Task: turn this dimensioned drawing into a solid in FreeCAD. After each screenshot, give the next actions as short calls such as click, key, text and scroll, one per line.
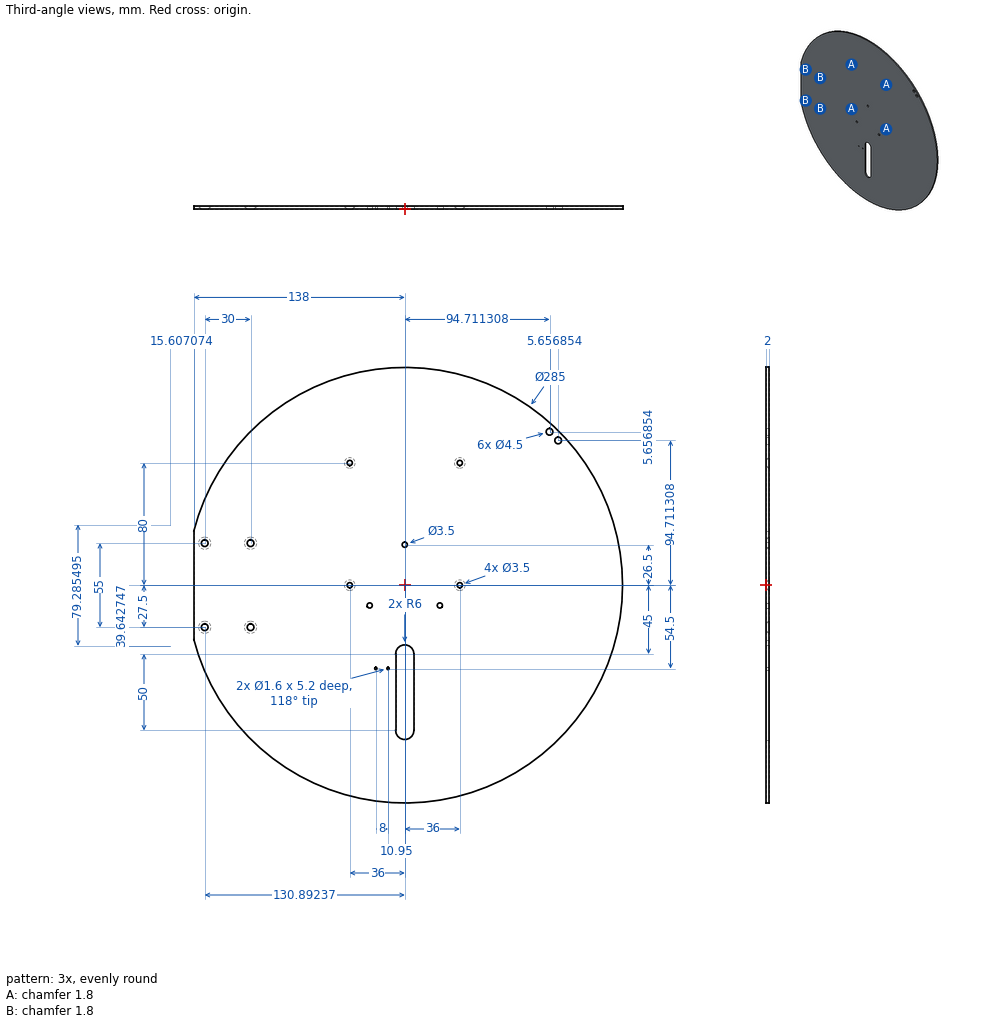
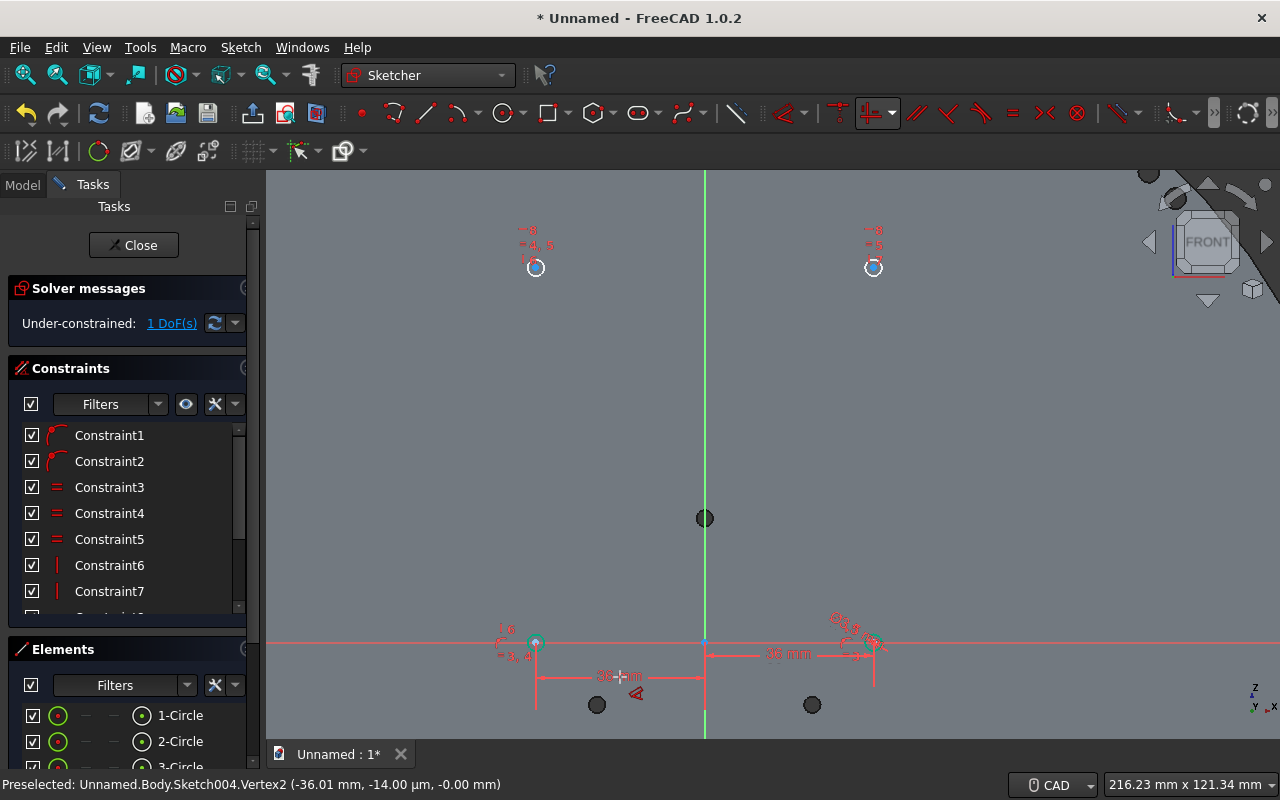
click(536, 268)
click(502, 455)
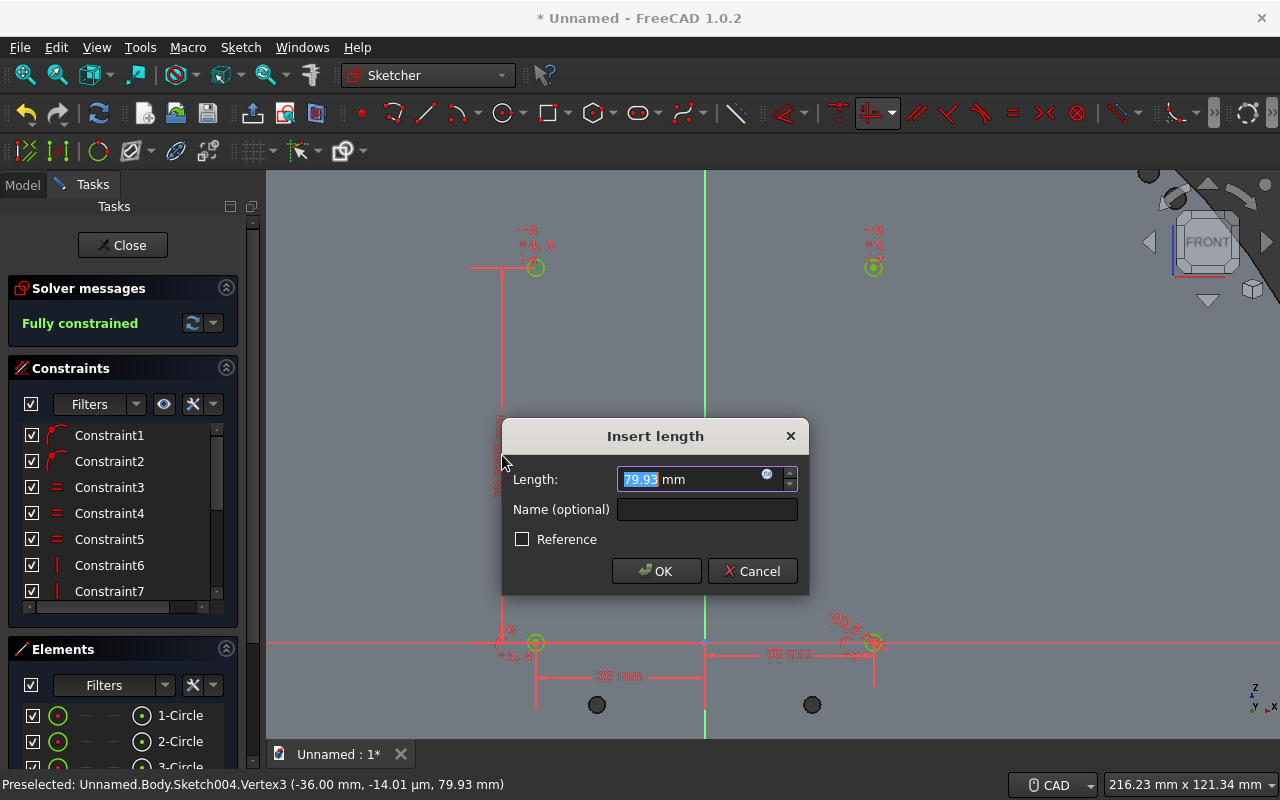
text(80)
key(Return)
key(Escape)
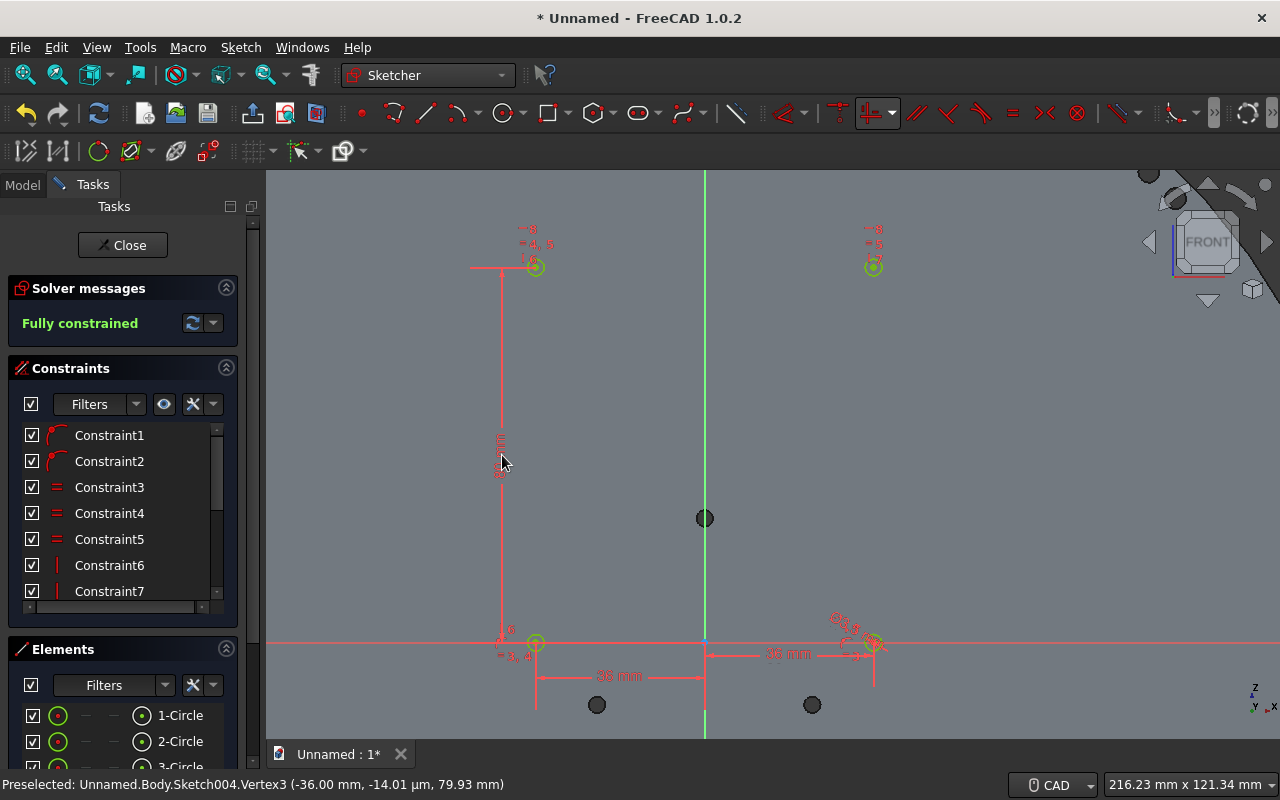
click(123, 245)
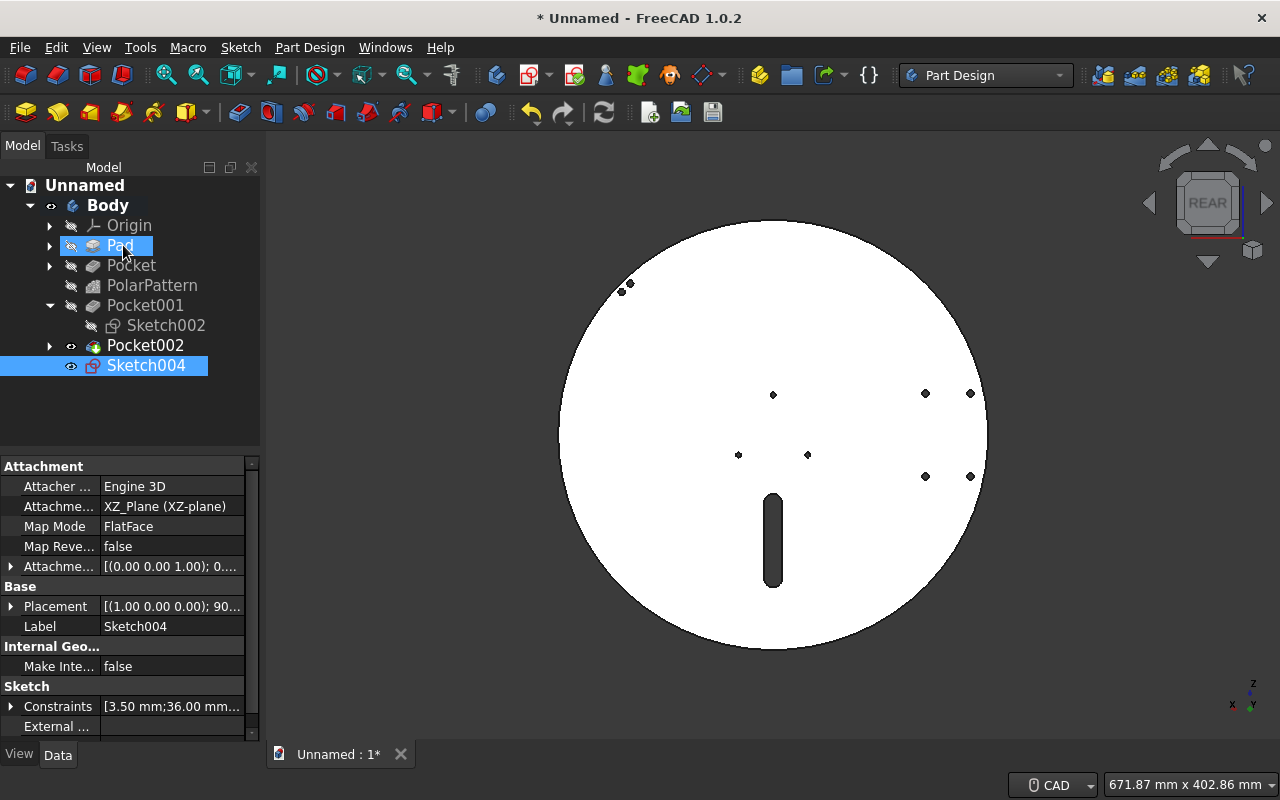
click(240, 112)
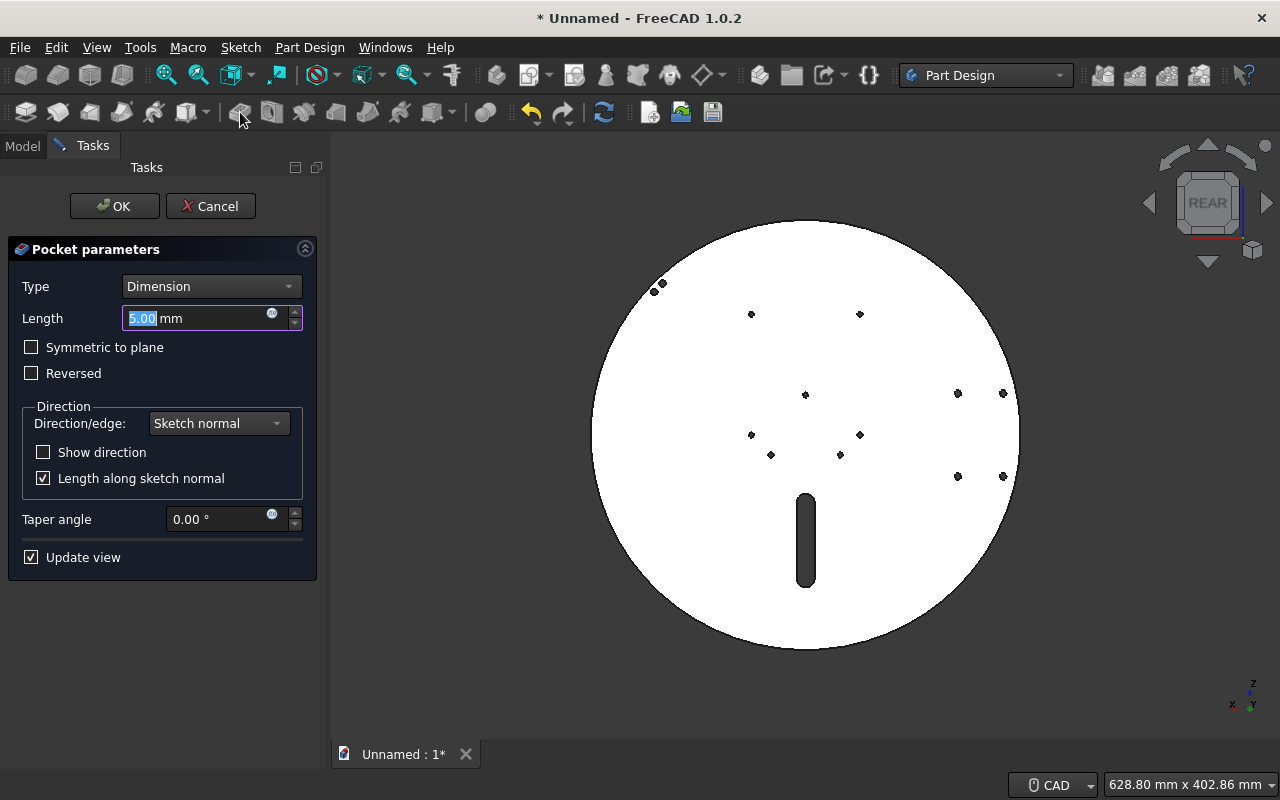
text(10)
key(Tab)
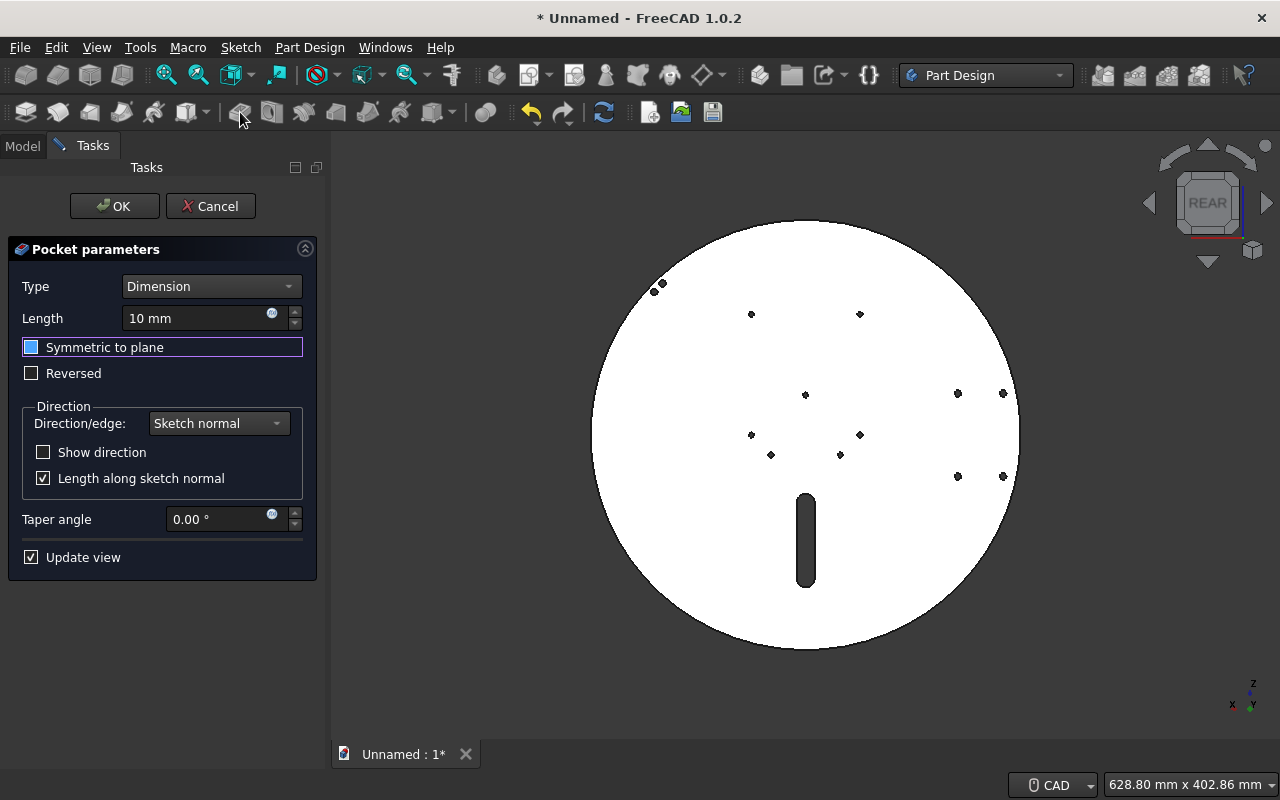
click(115, 206)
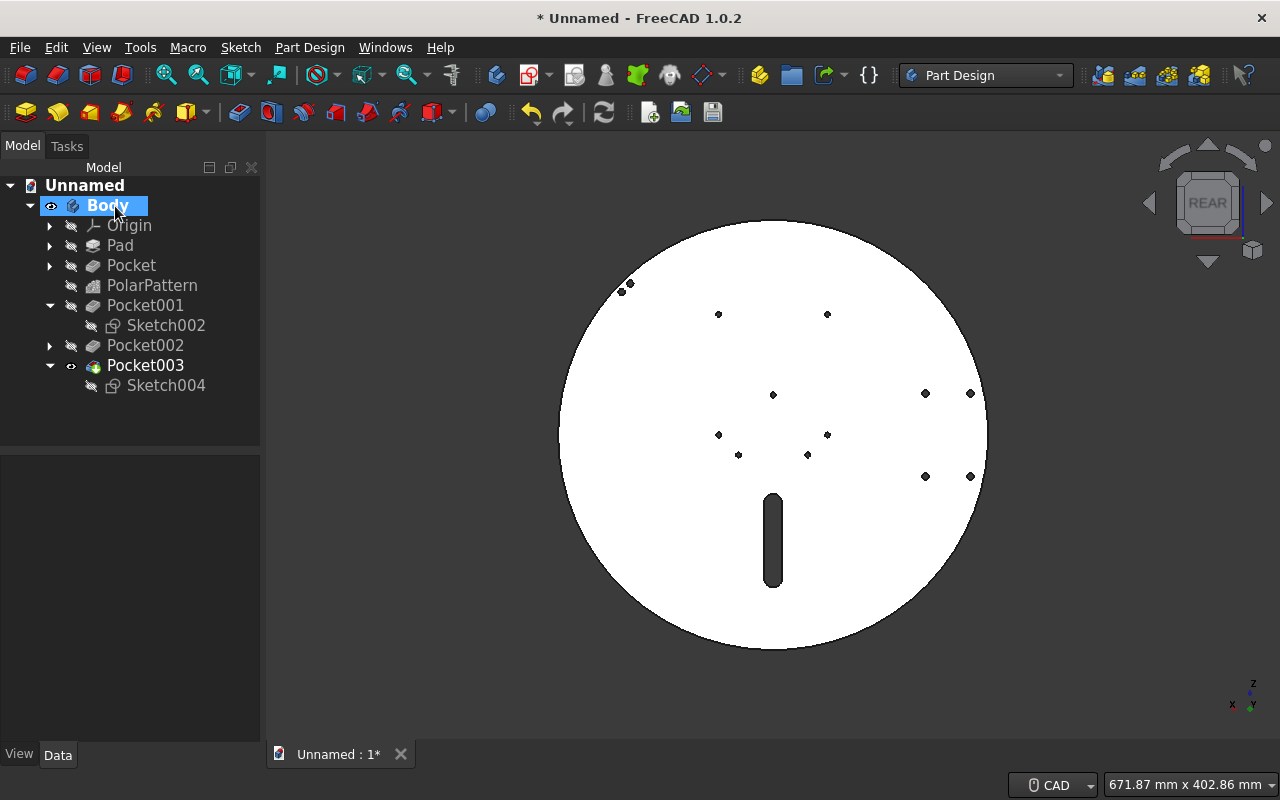
click(721, 434)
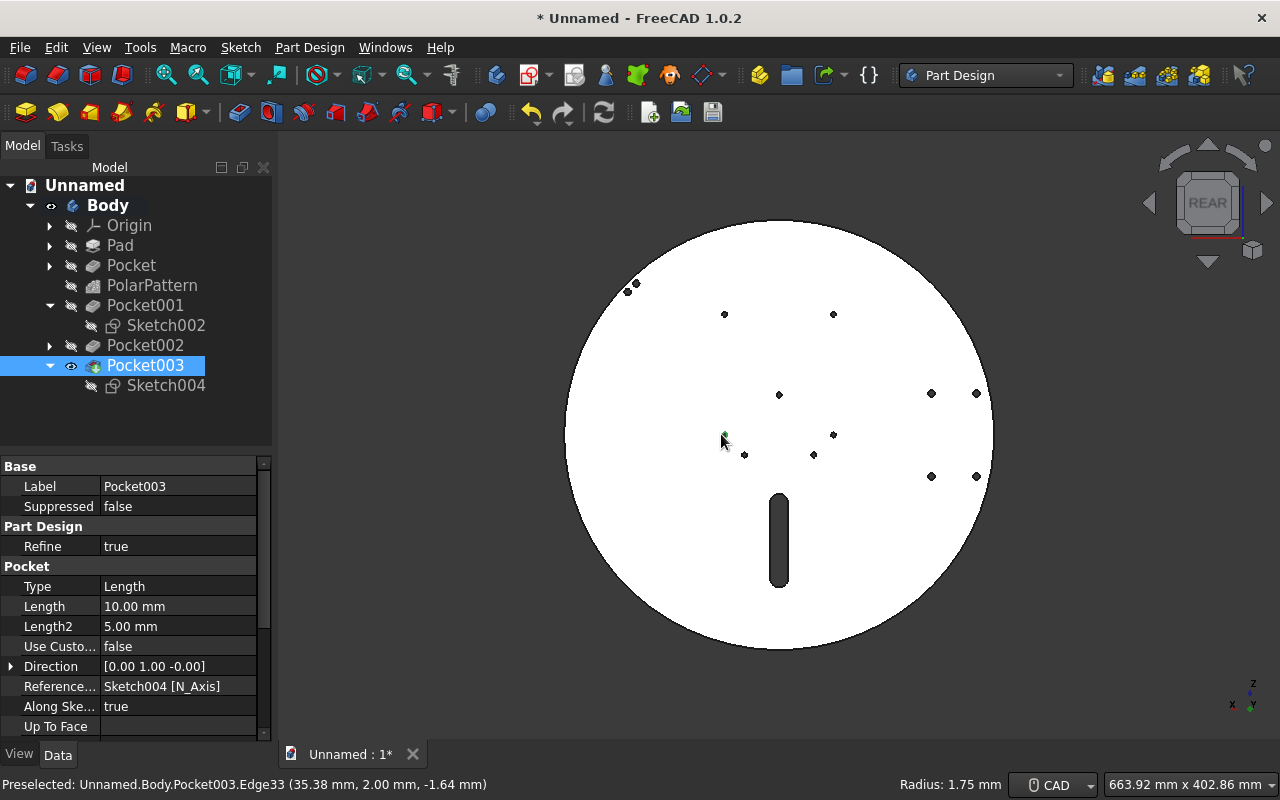
click(836, 434, ctrl)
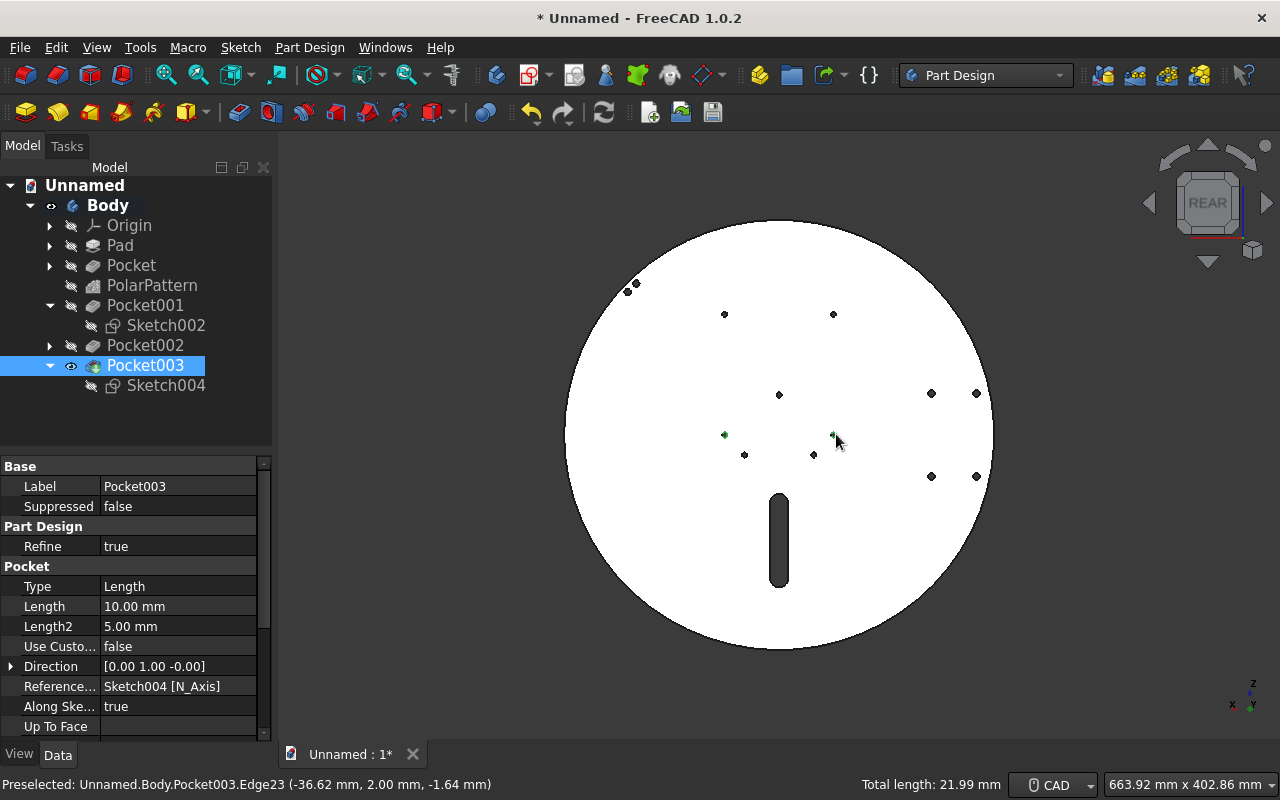
click(836, 313, ctrl)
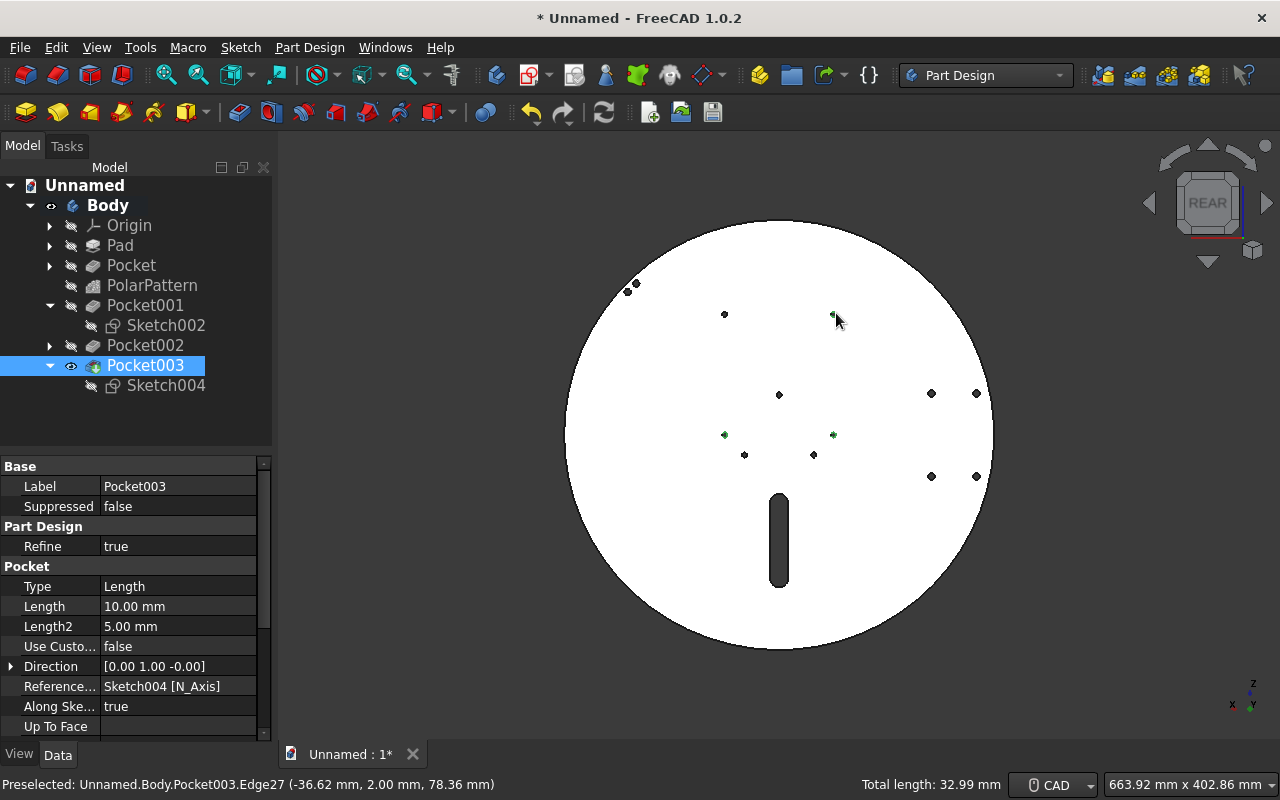
click(727, 313, ctrl)